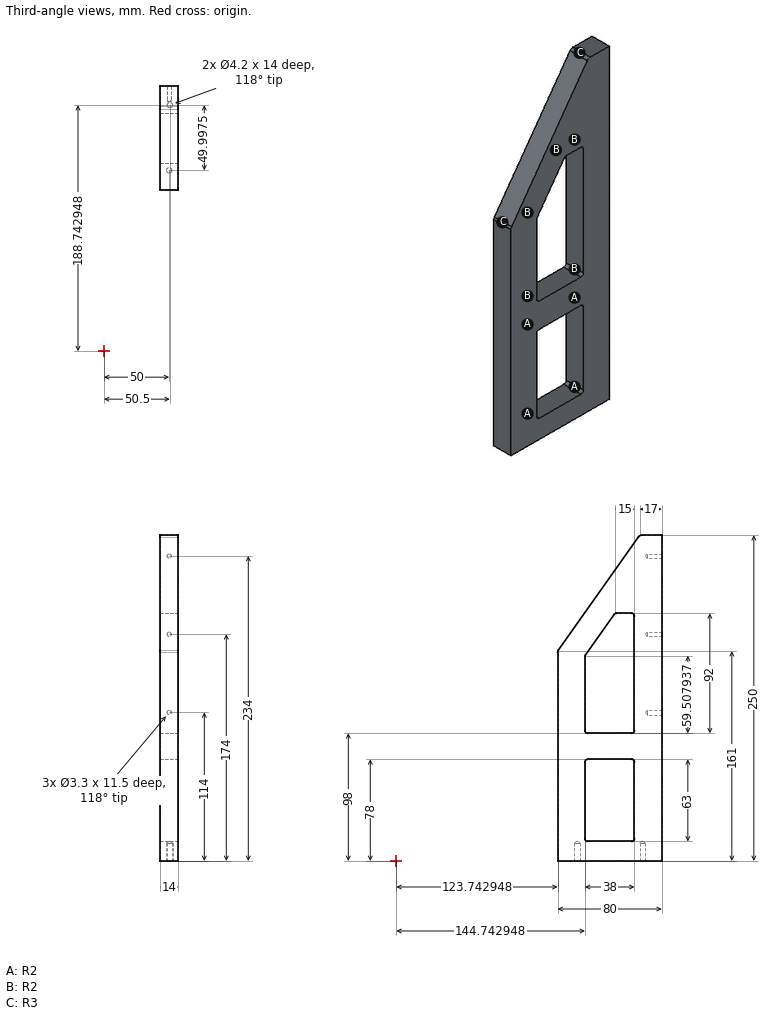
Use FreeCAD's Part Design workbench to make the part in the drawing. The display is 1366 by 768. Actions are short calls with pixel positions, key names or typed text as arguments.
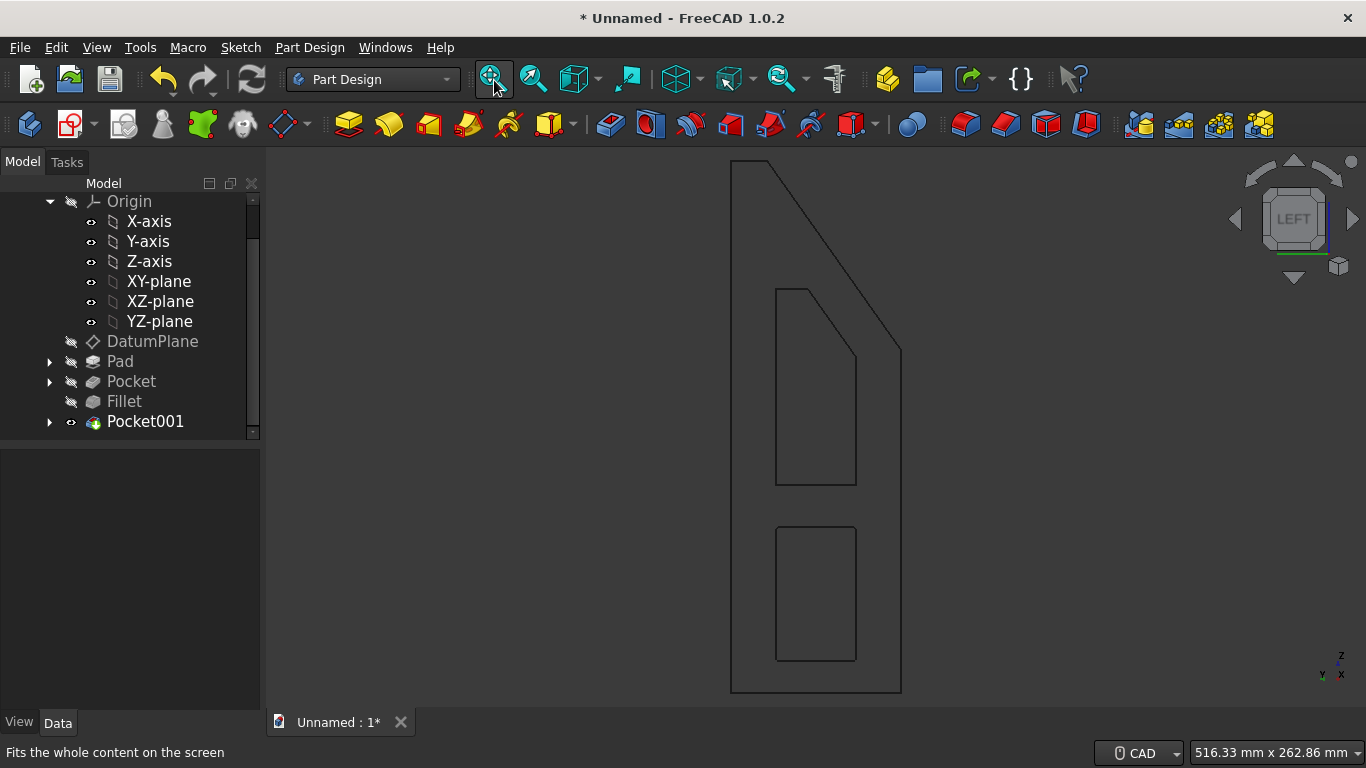
key(0)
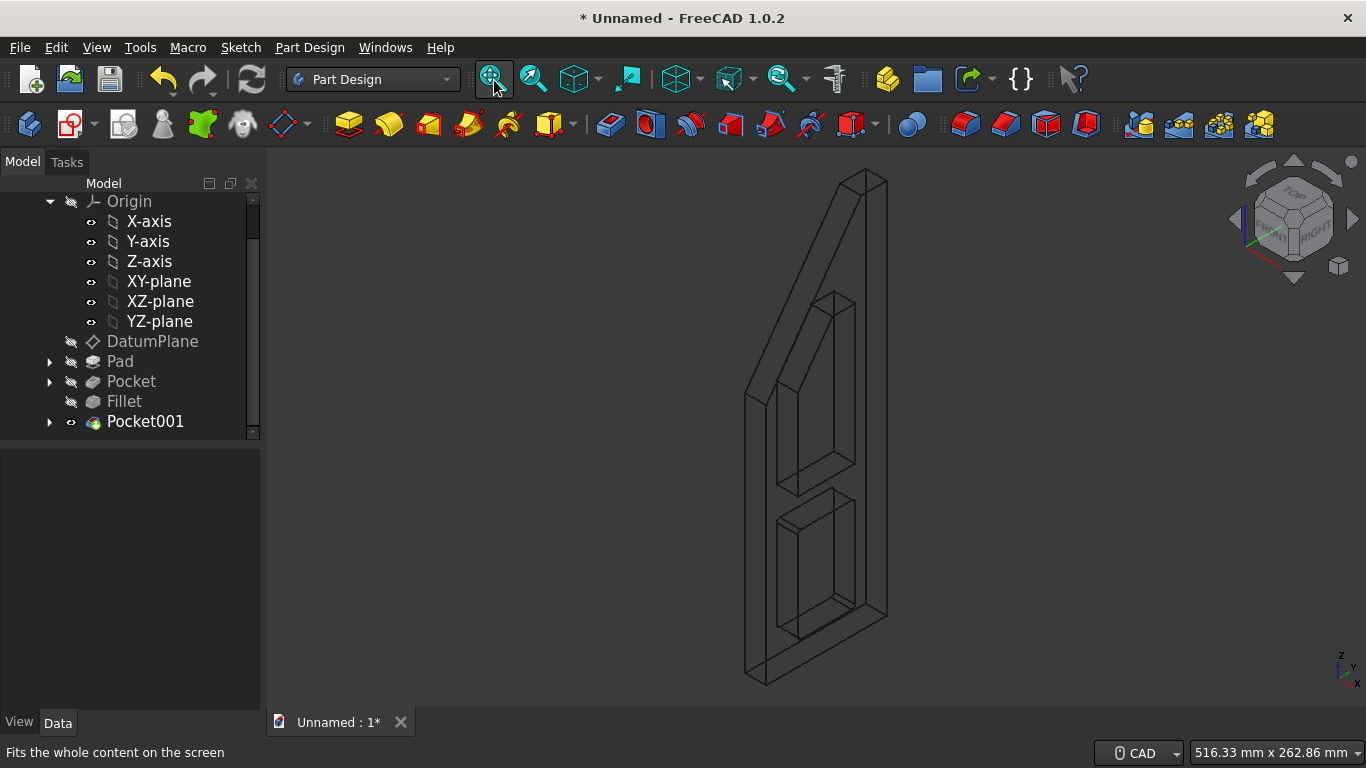
click(845, 456)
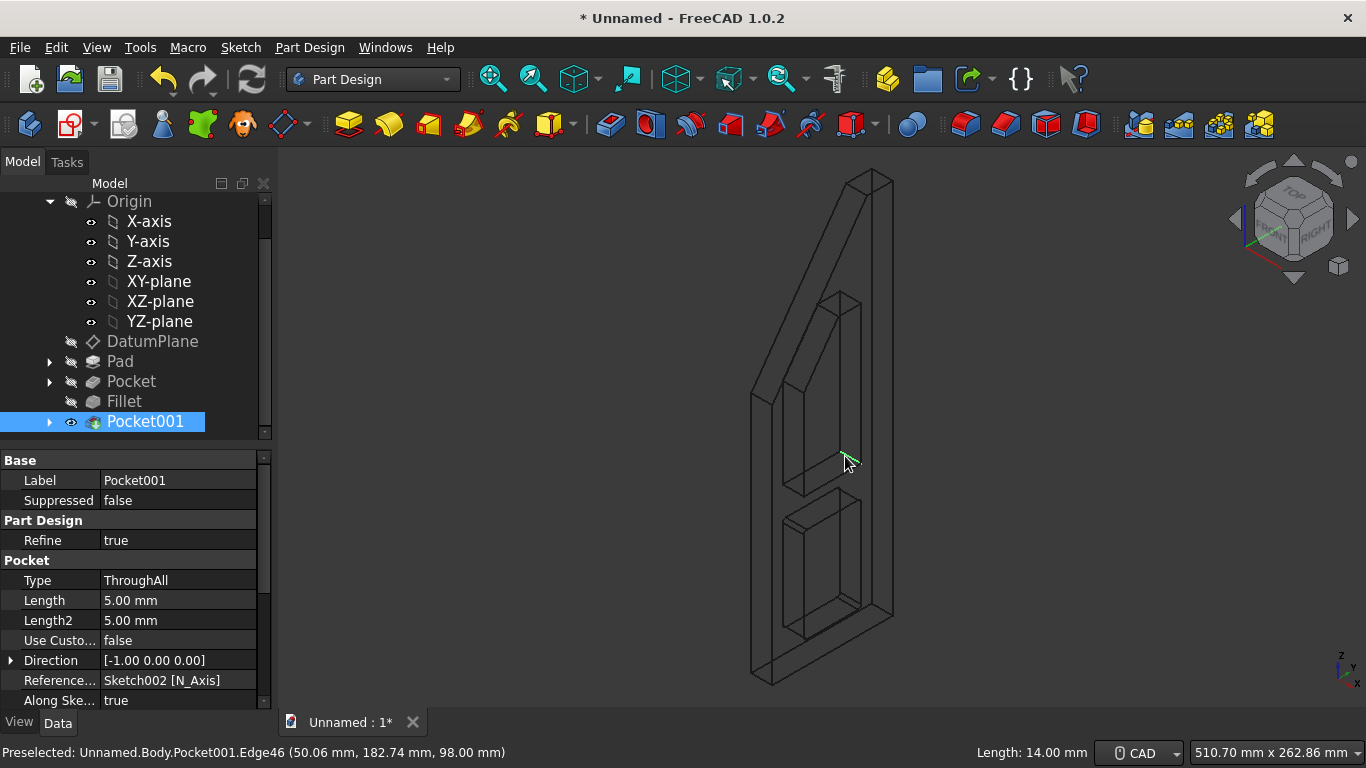
click(793, 489, ctrl)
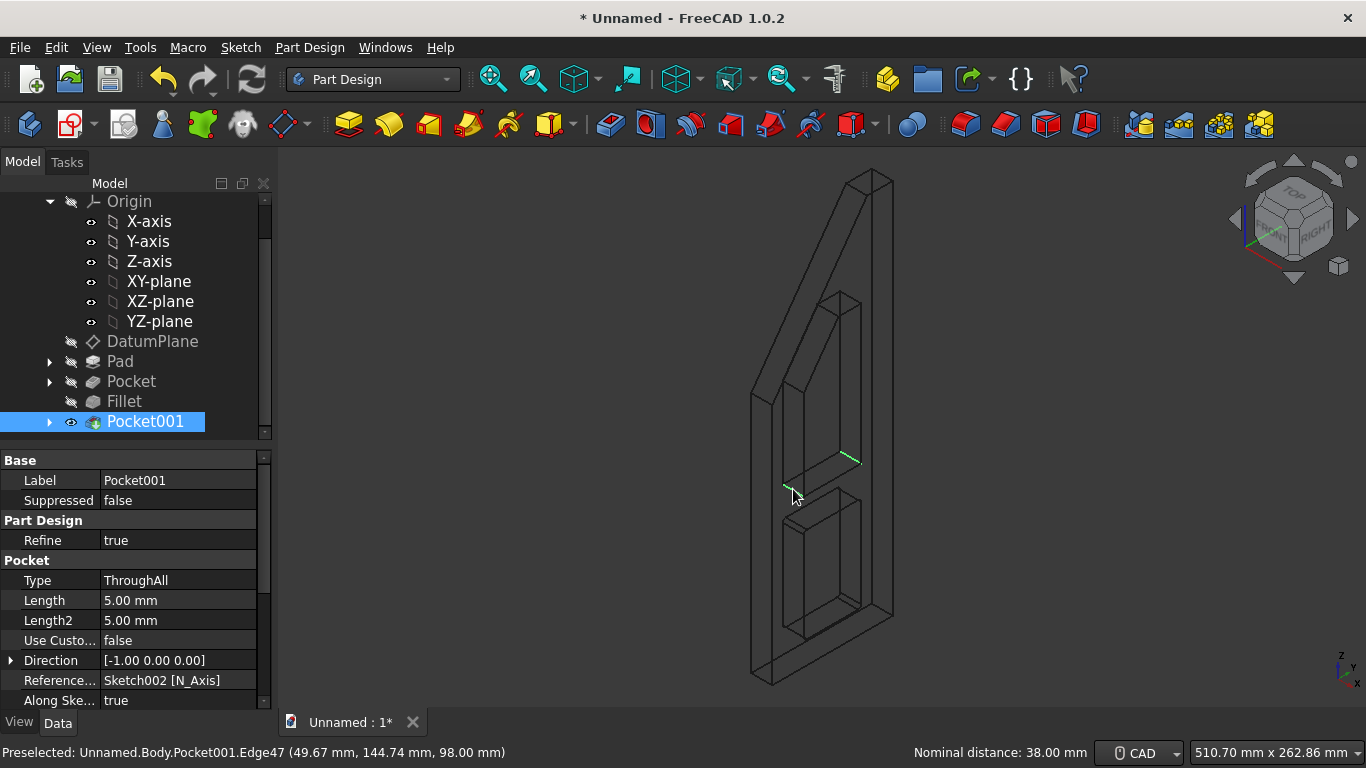
click(793, 386, ctrl)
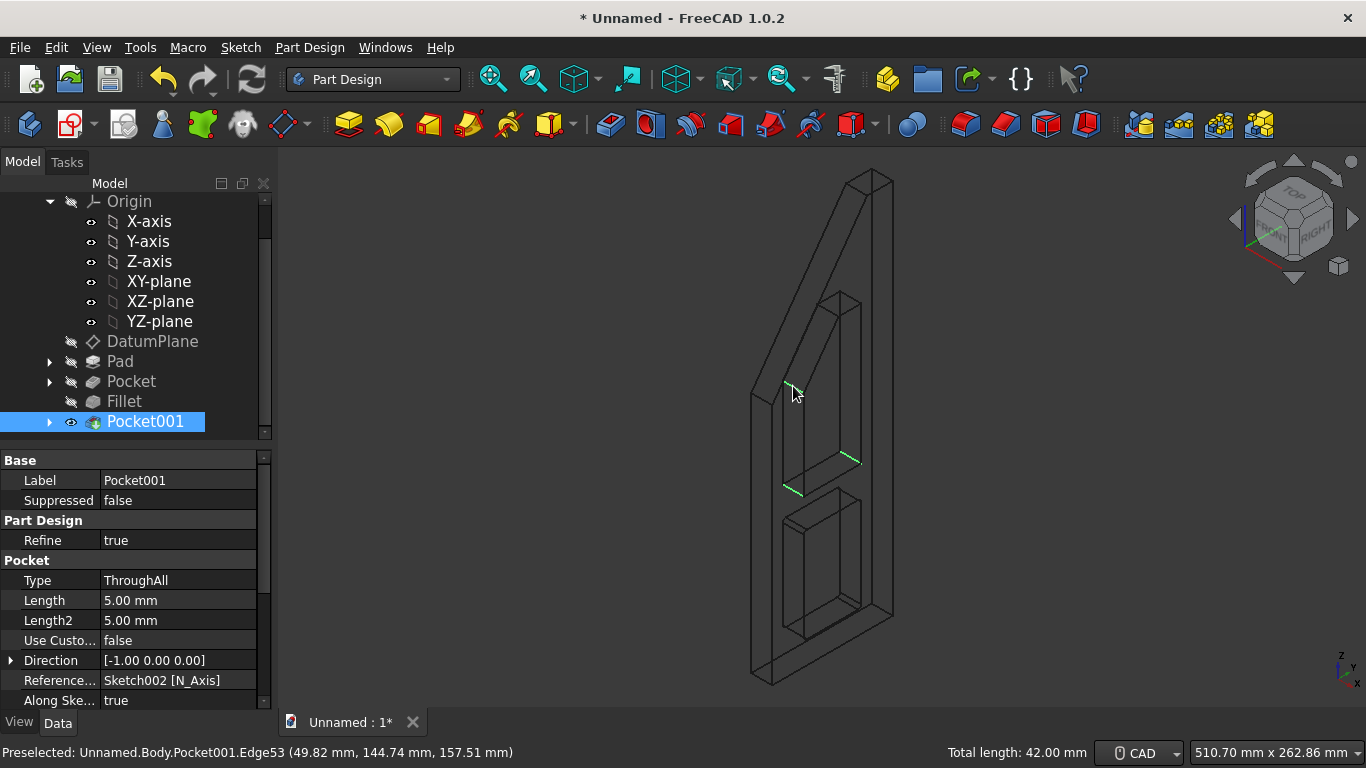
click(828, 309, ctrl)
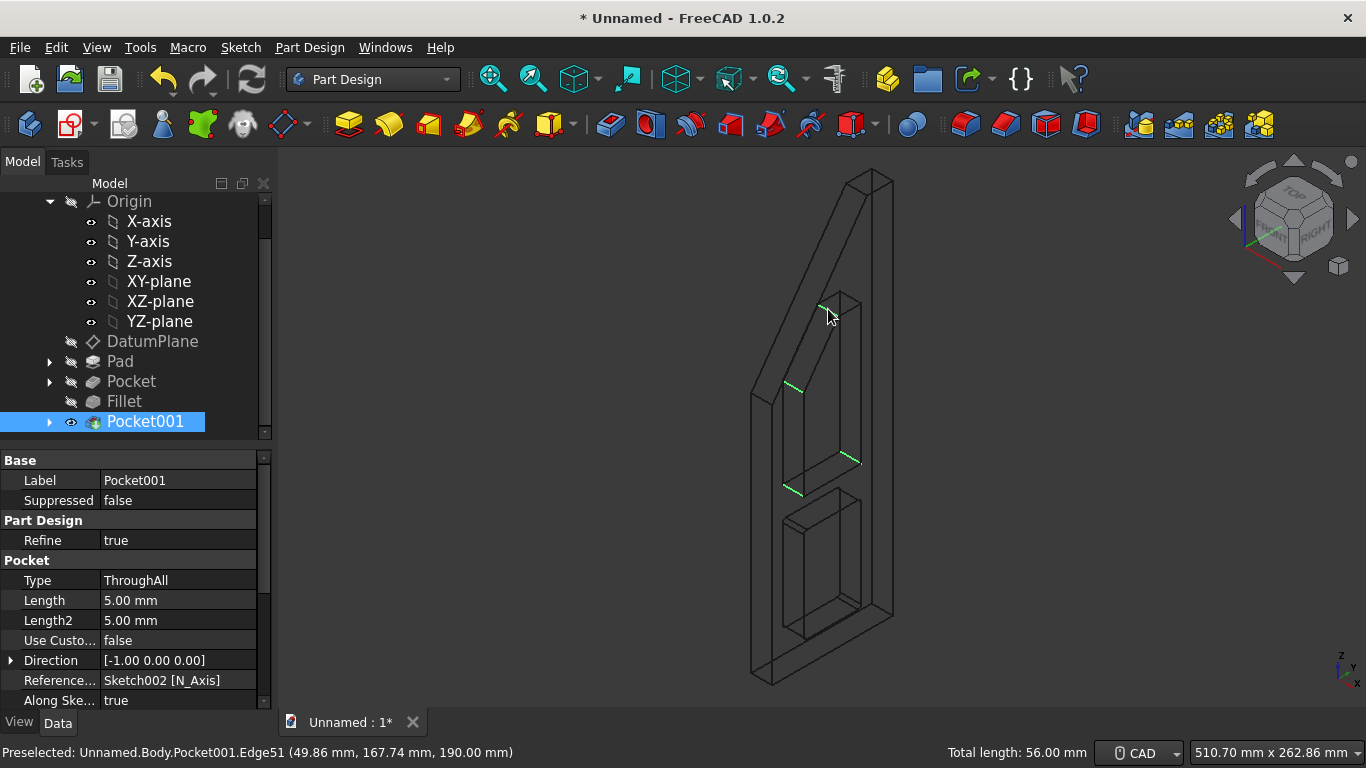
click(851, 296, ctrl)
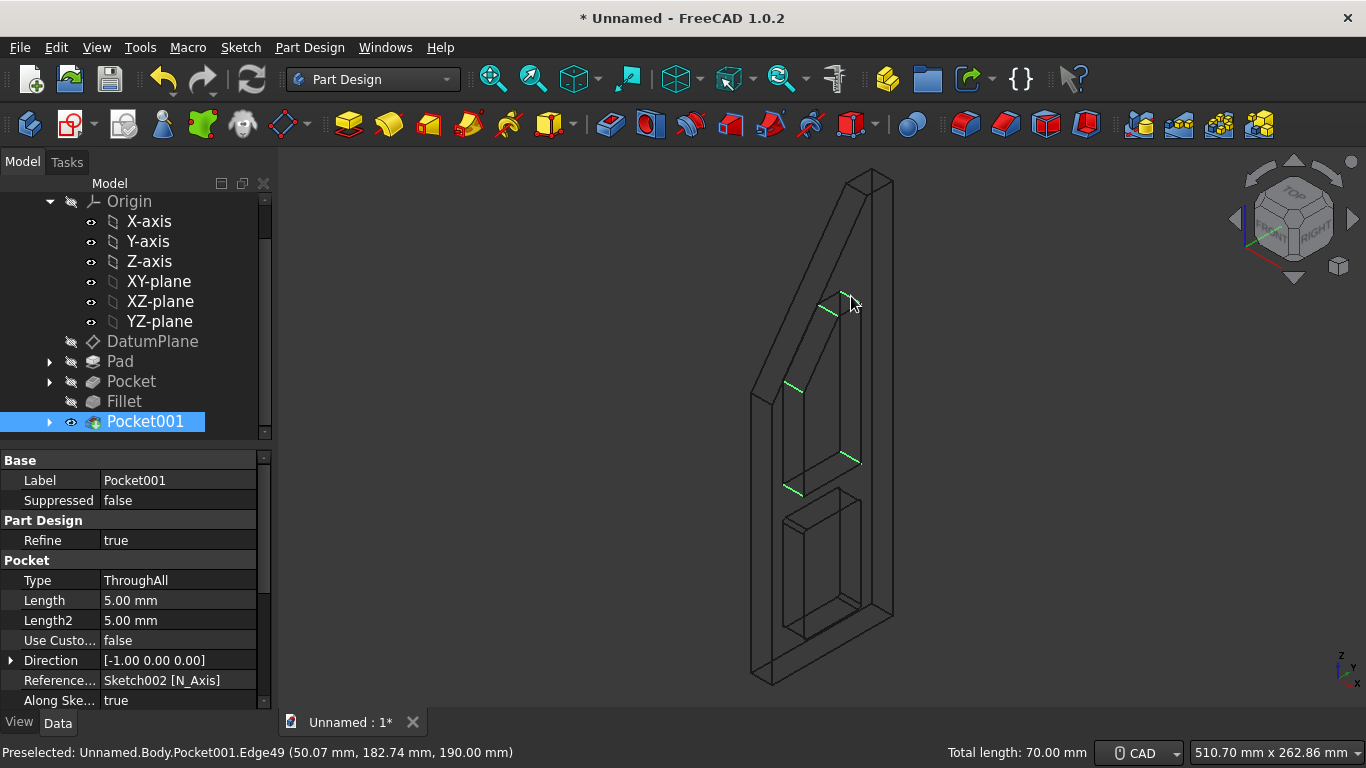
key(v)
key(1)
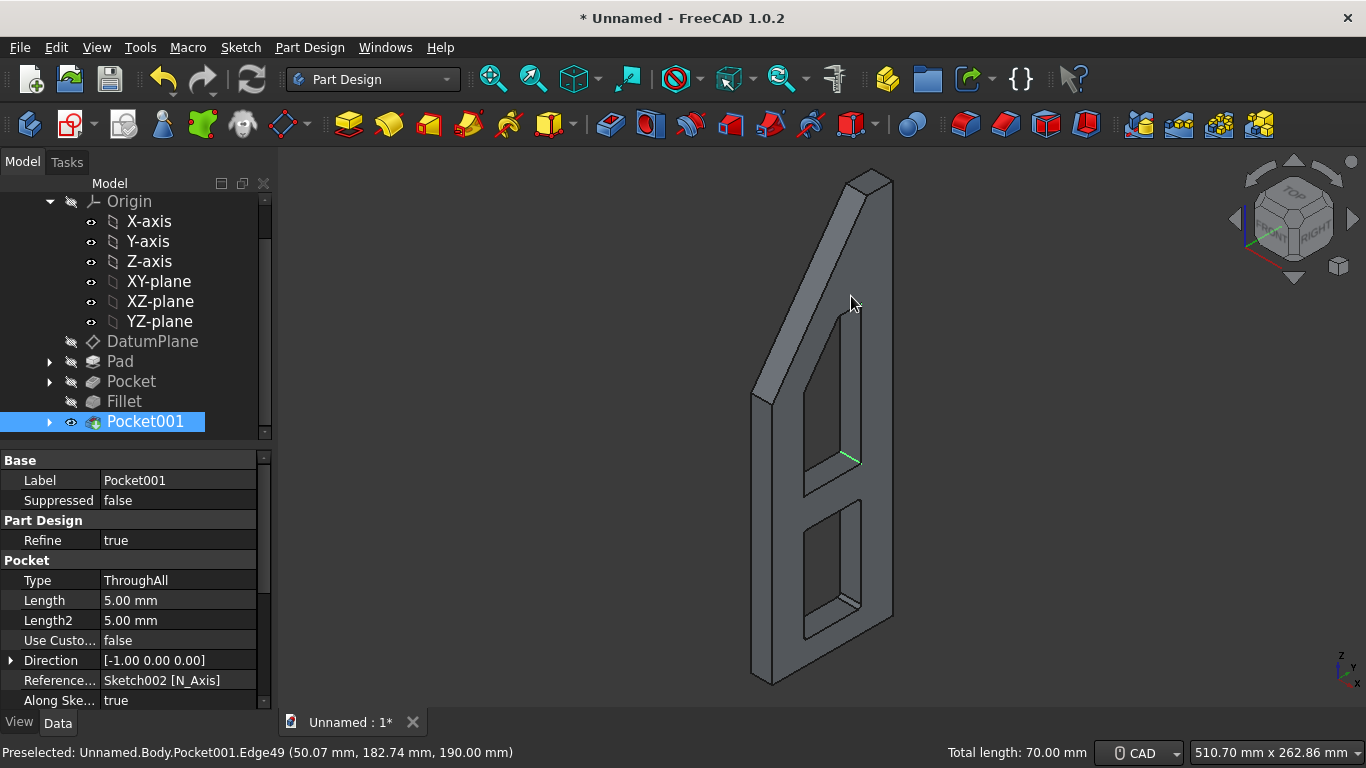
click(966, 124)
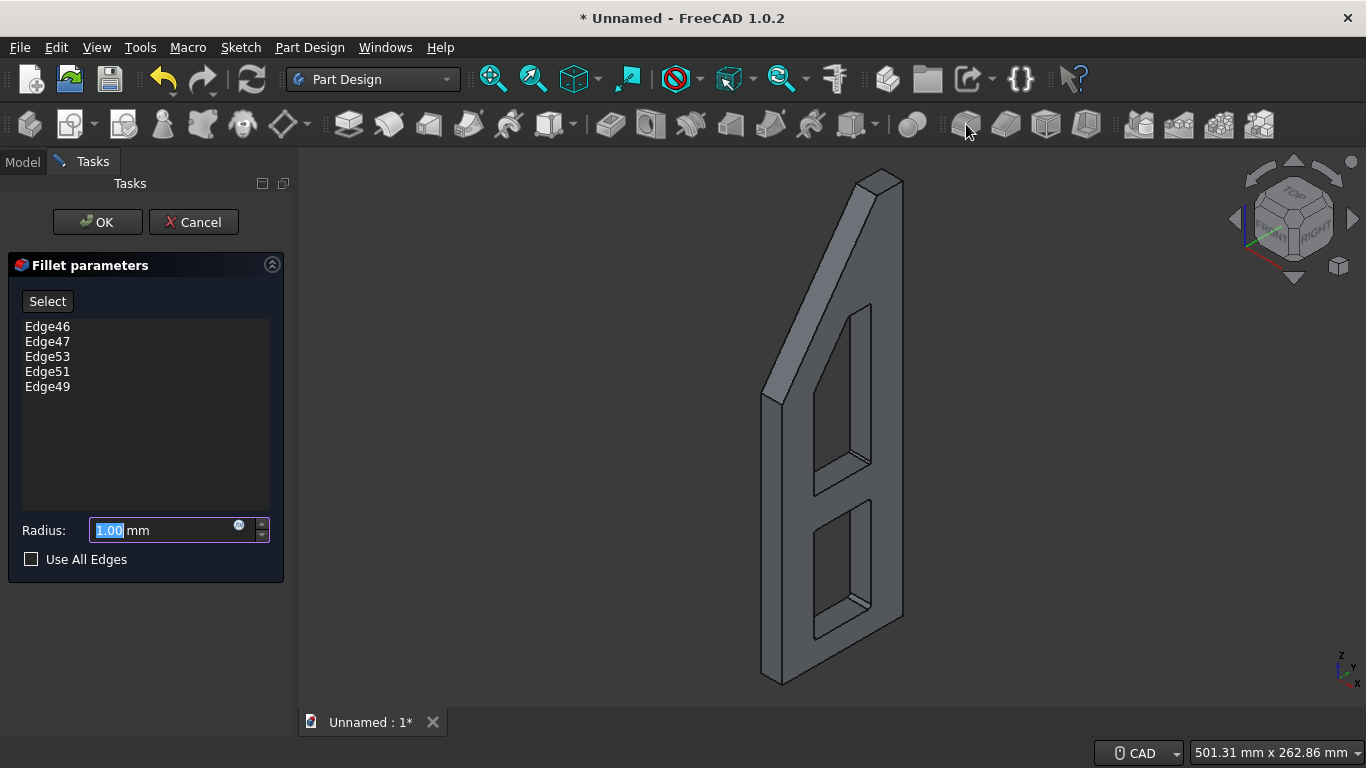
text(2)
key(Tab)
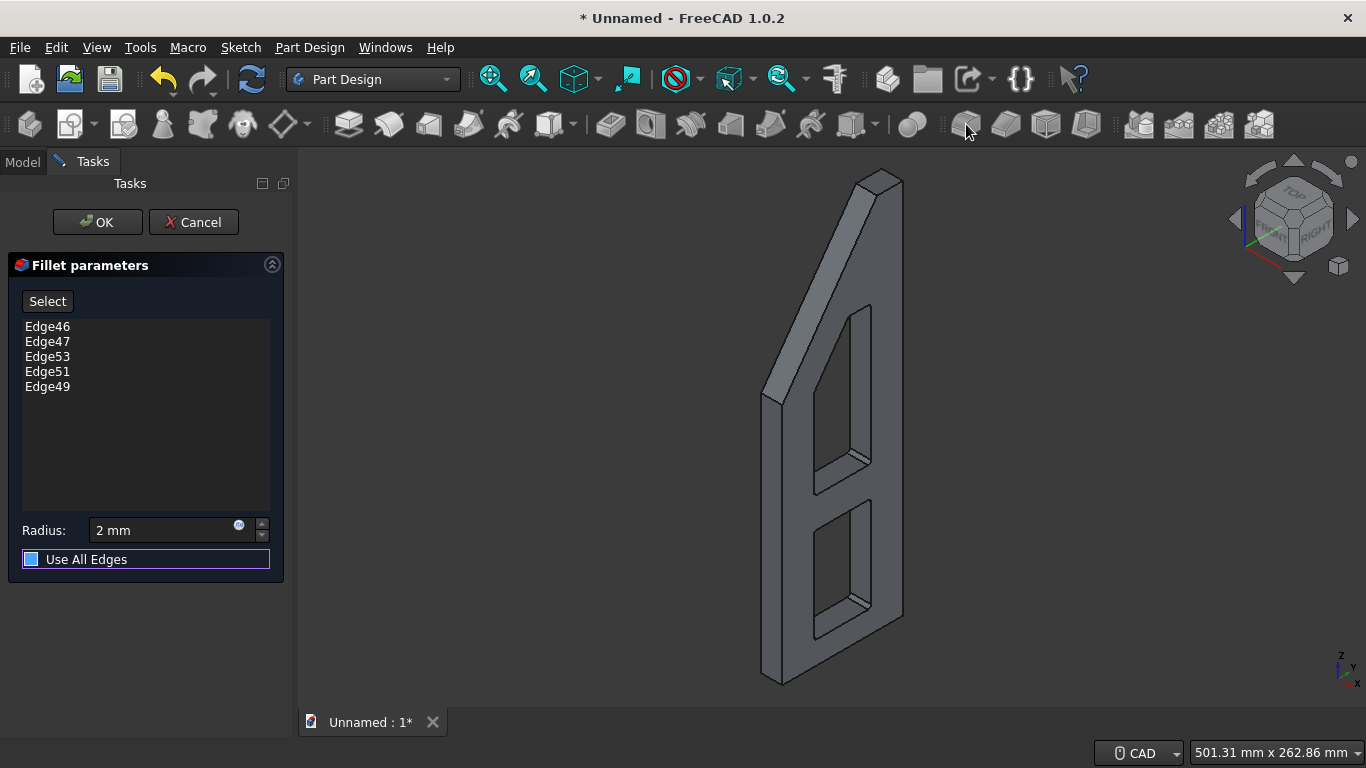
click(98, 222)